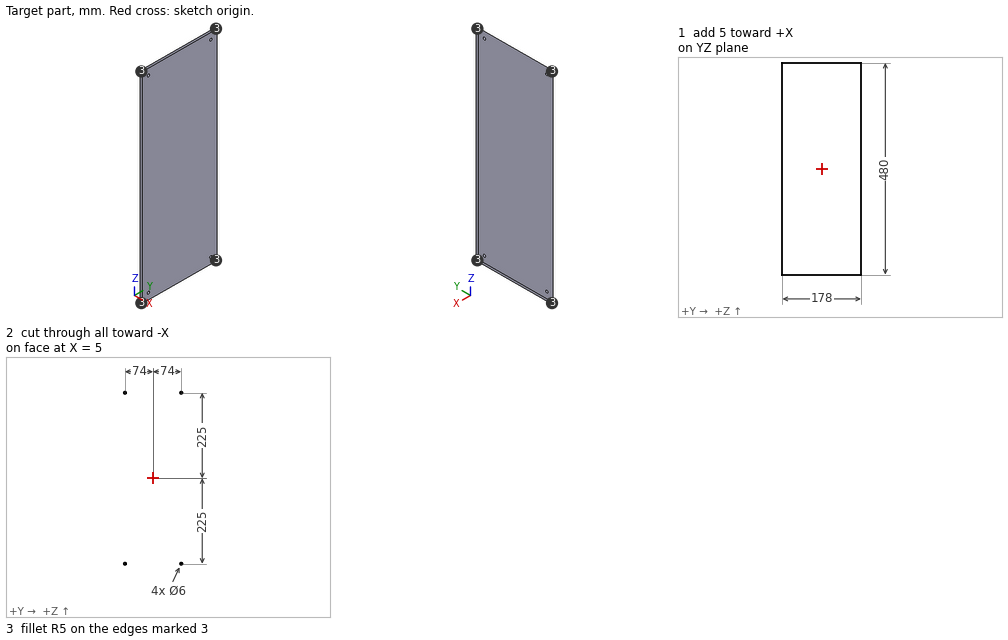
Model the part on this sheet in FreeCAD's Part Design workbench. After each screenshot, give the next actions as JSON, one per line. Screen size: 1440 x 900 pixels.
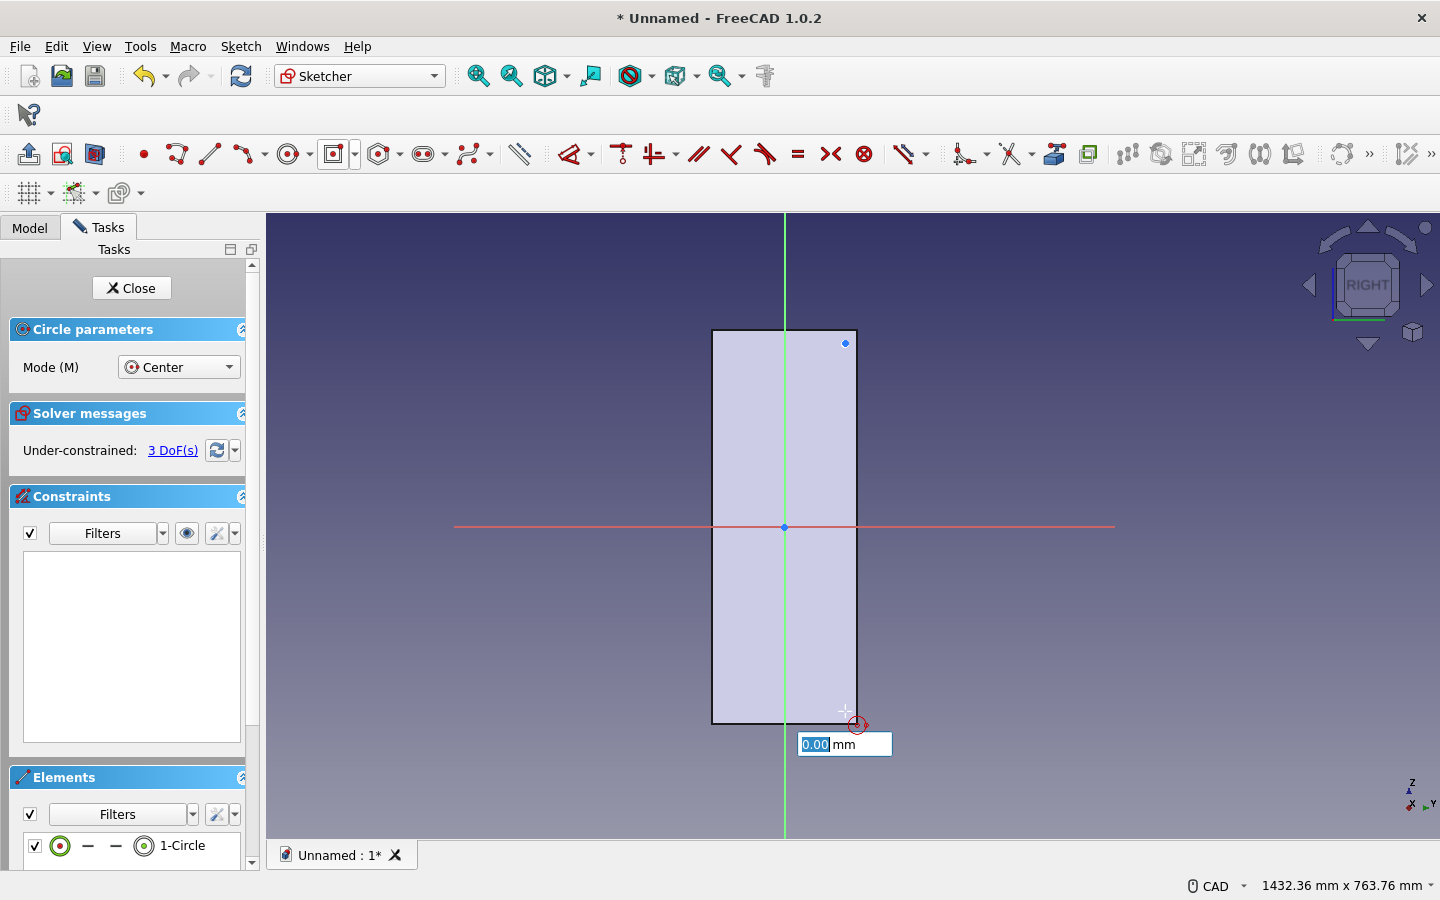
{"action": "scroll", "coordinate": [847, 710], "scroll_direction": "up", "scroll_amount": 10}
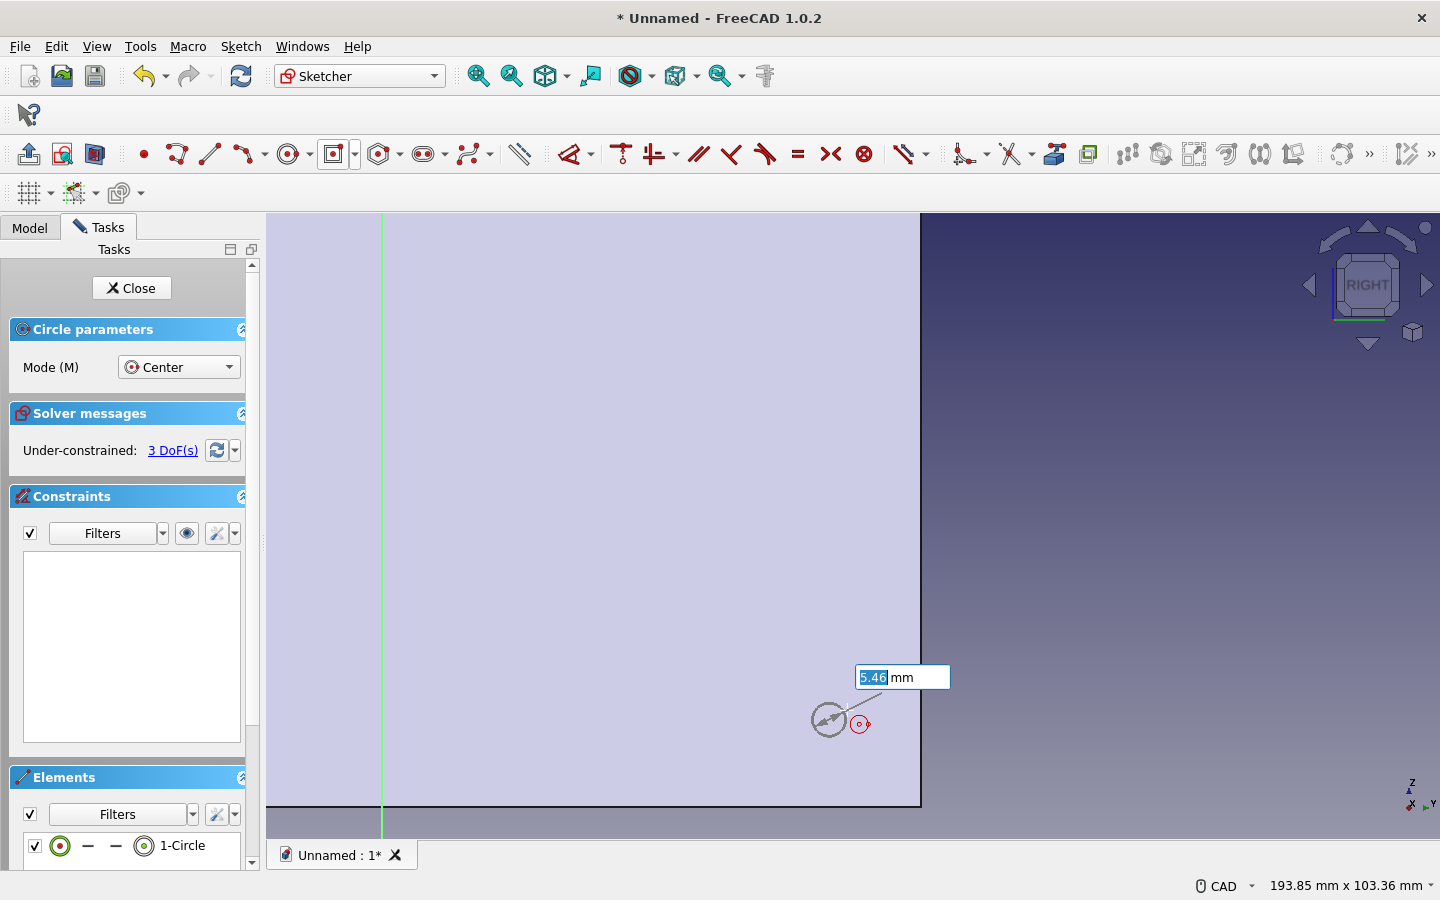
{"action": "left_click", "coordinate": [843, 703]}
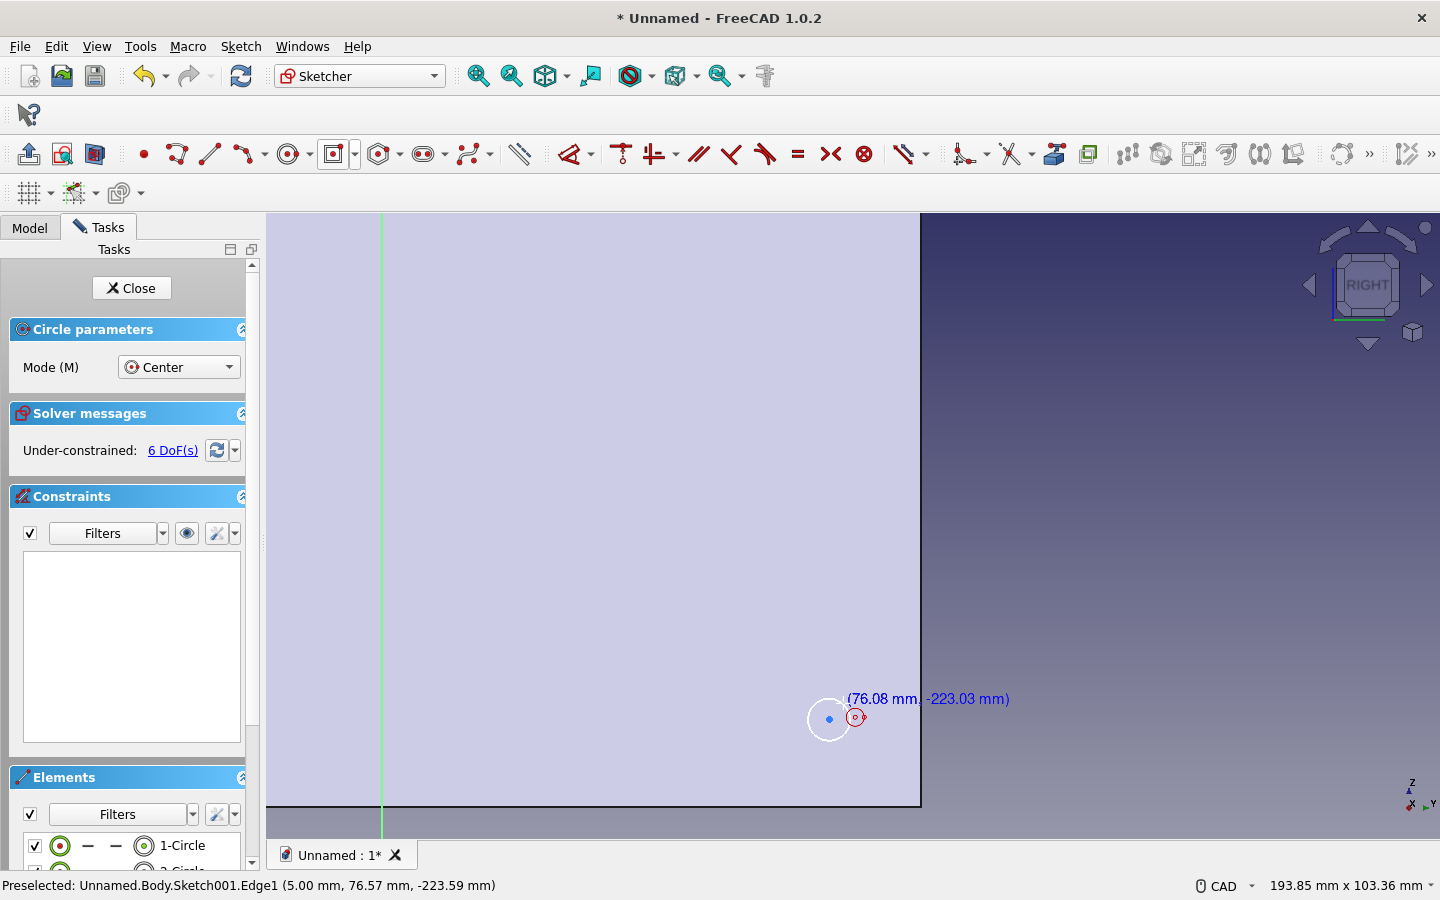
{"action": "scroll", "coordinate": [847, 710], "scroll_direction": "down", "scroll_amount": 10}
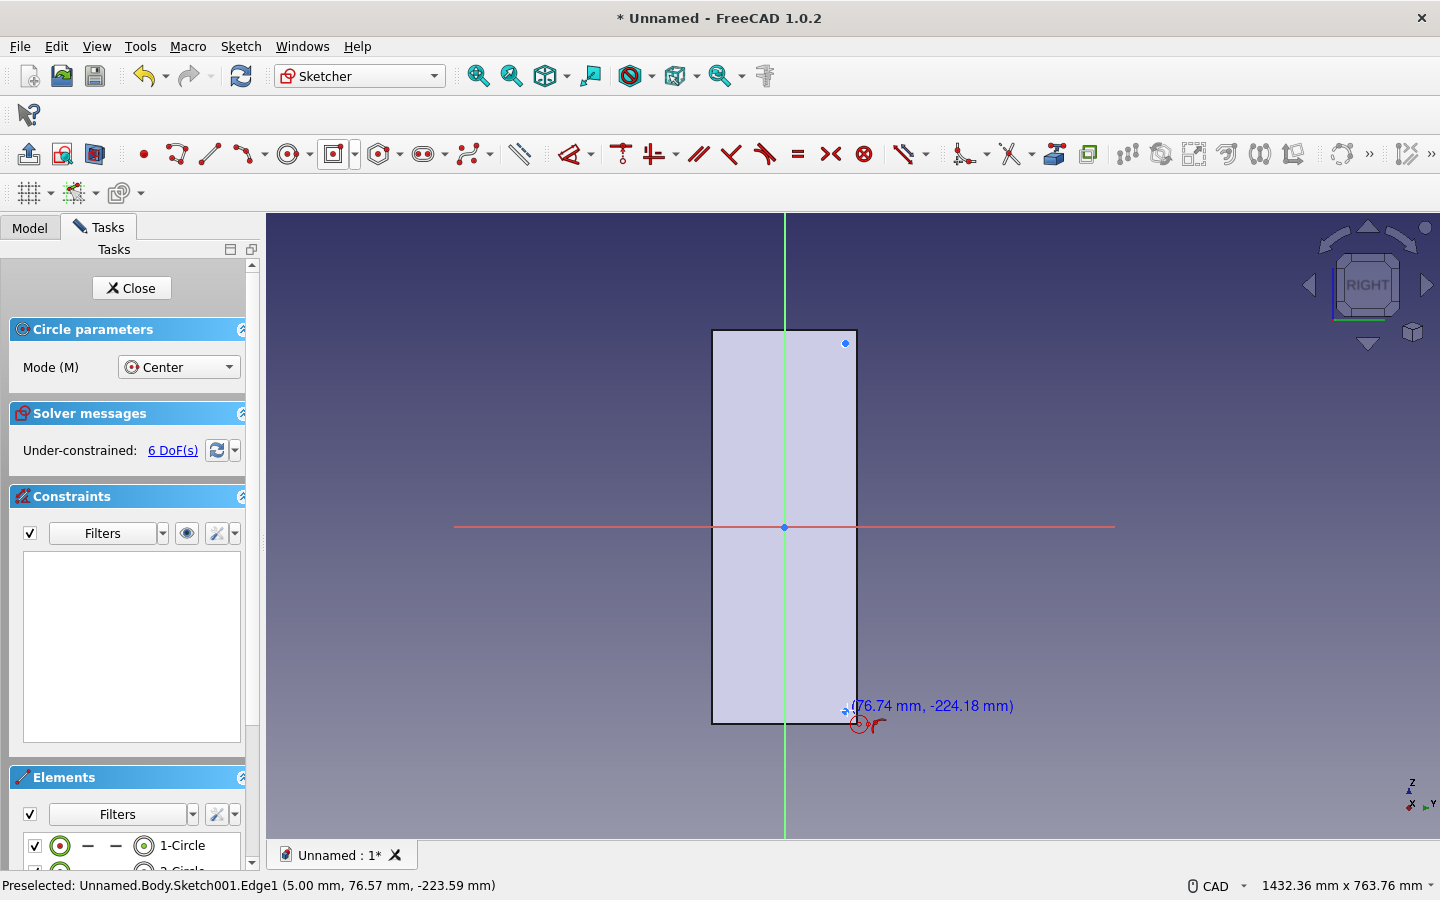
{"action": "scroll", "coordinate": [724, 343], "scroll_direction": "up", "scroll_amount": 12}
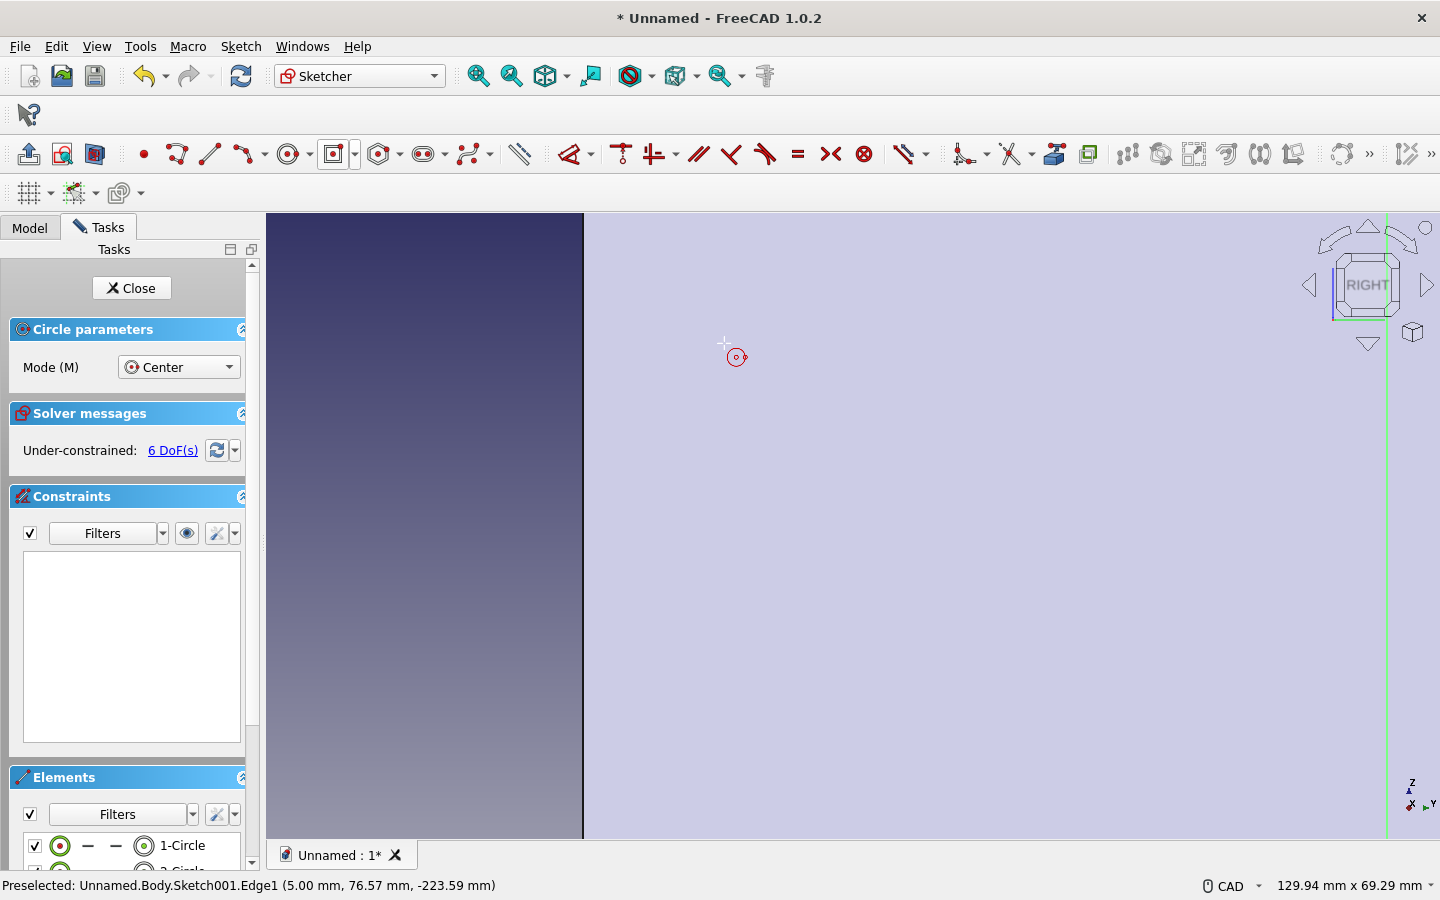
{"action": "scroll", "coordinate": [724, 342], "scroll_direction": "down", "scroll_amount": 12}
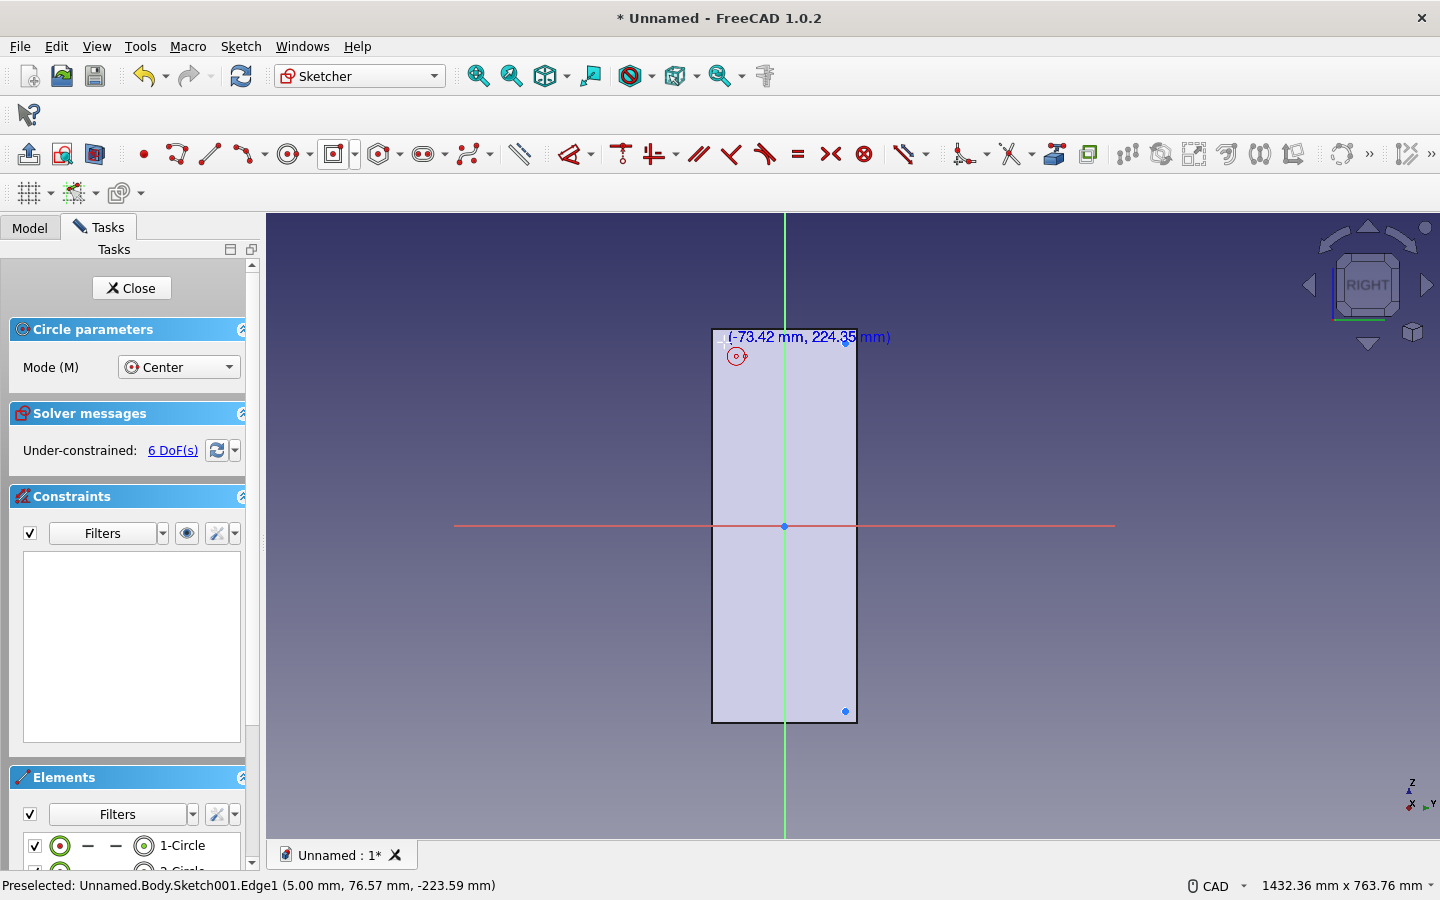
{"action": "left_click", "coordinate": [724, 342]}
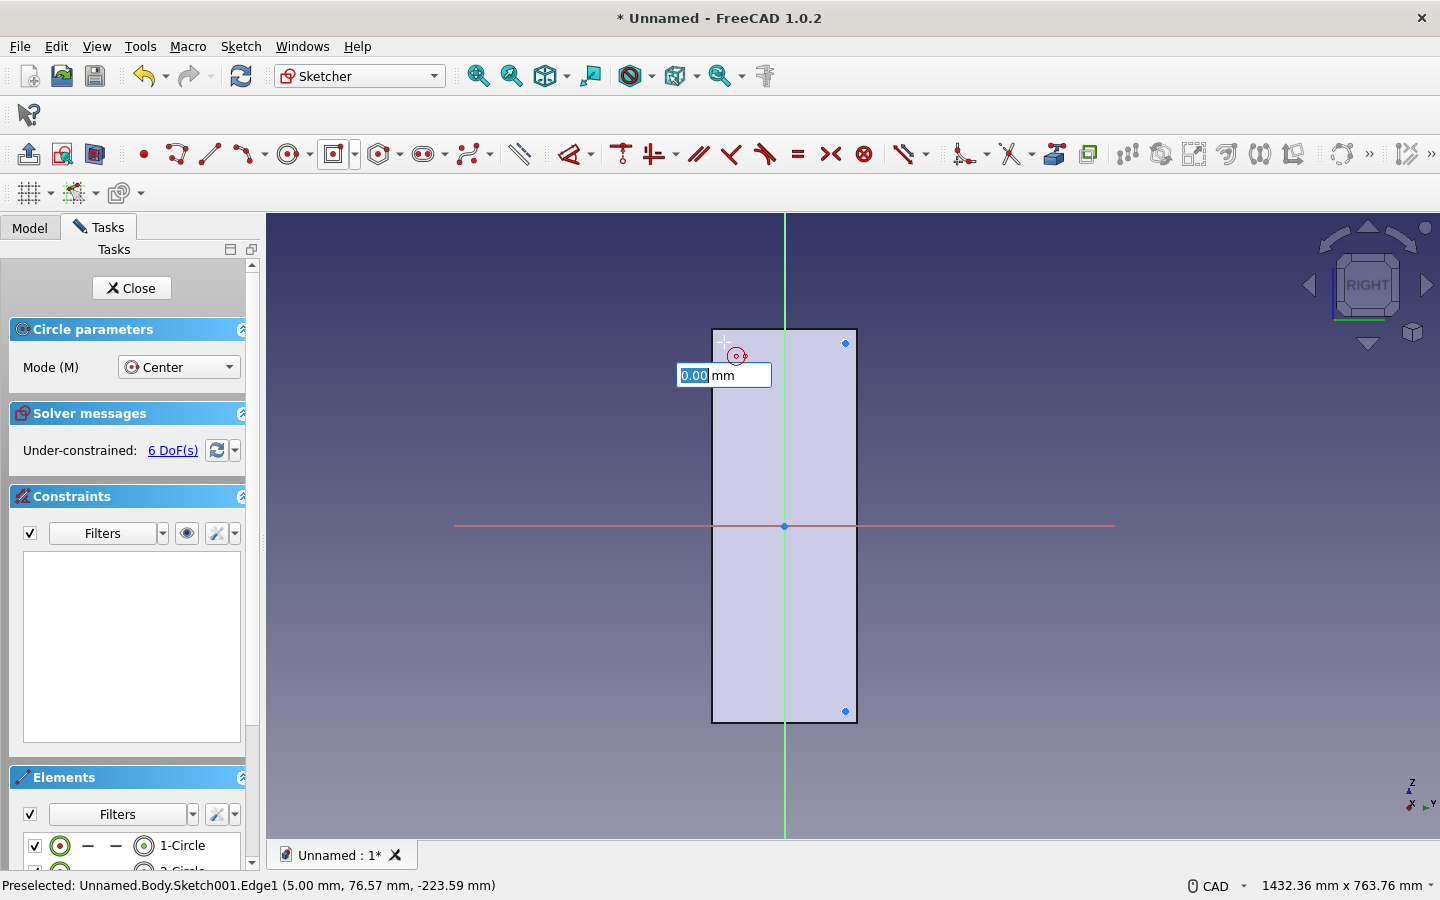
{"action": "scroll", "coordinate": [726, 340], "scroll_direction": "up", "scroll_amount": 10}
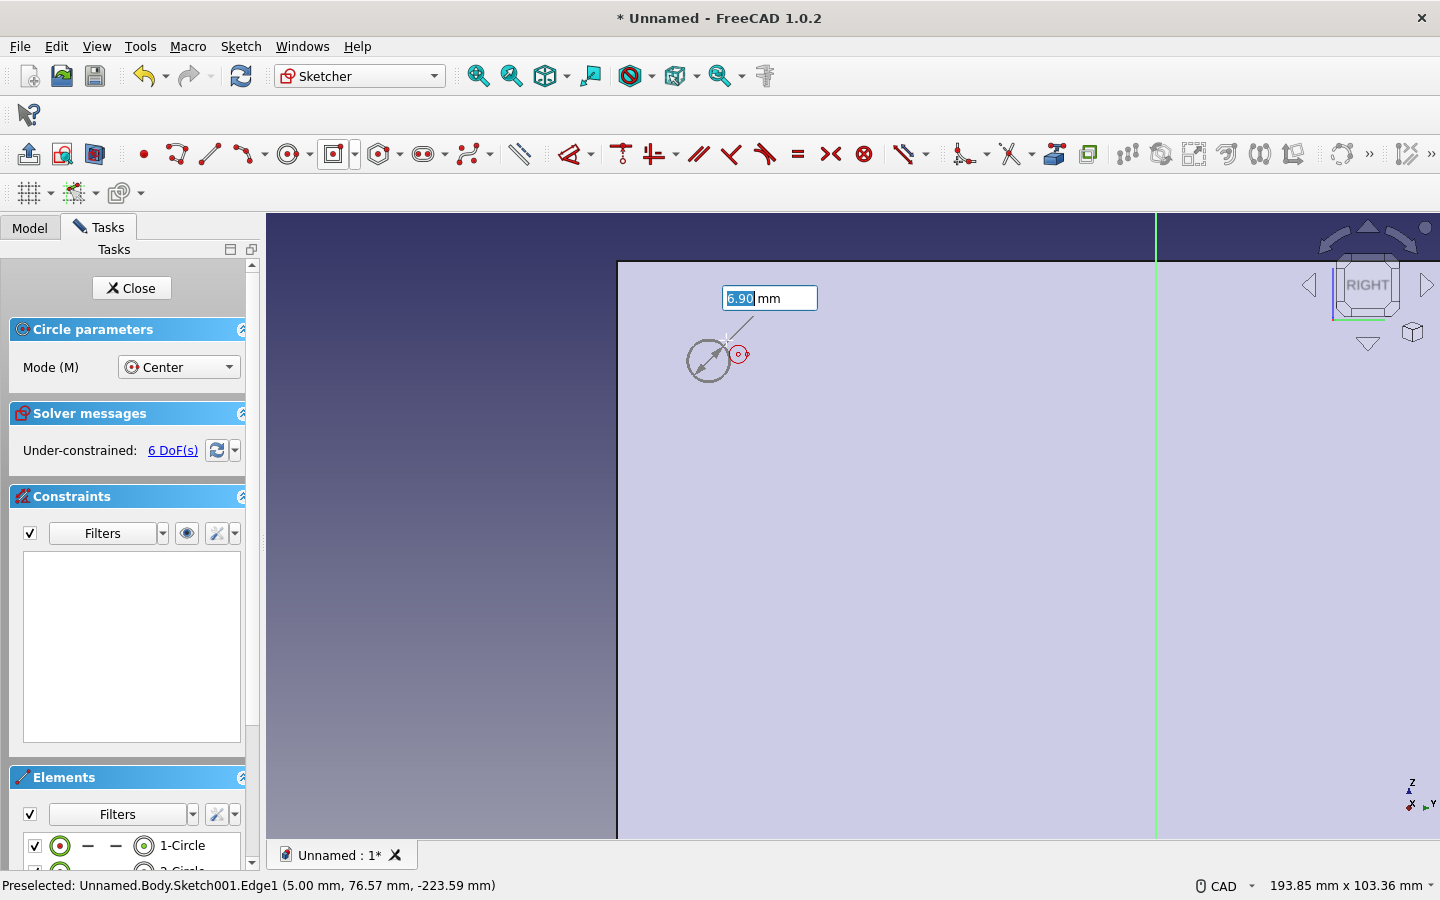
{"action": "left_click", "coordinate": [721, 339]}